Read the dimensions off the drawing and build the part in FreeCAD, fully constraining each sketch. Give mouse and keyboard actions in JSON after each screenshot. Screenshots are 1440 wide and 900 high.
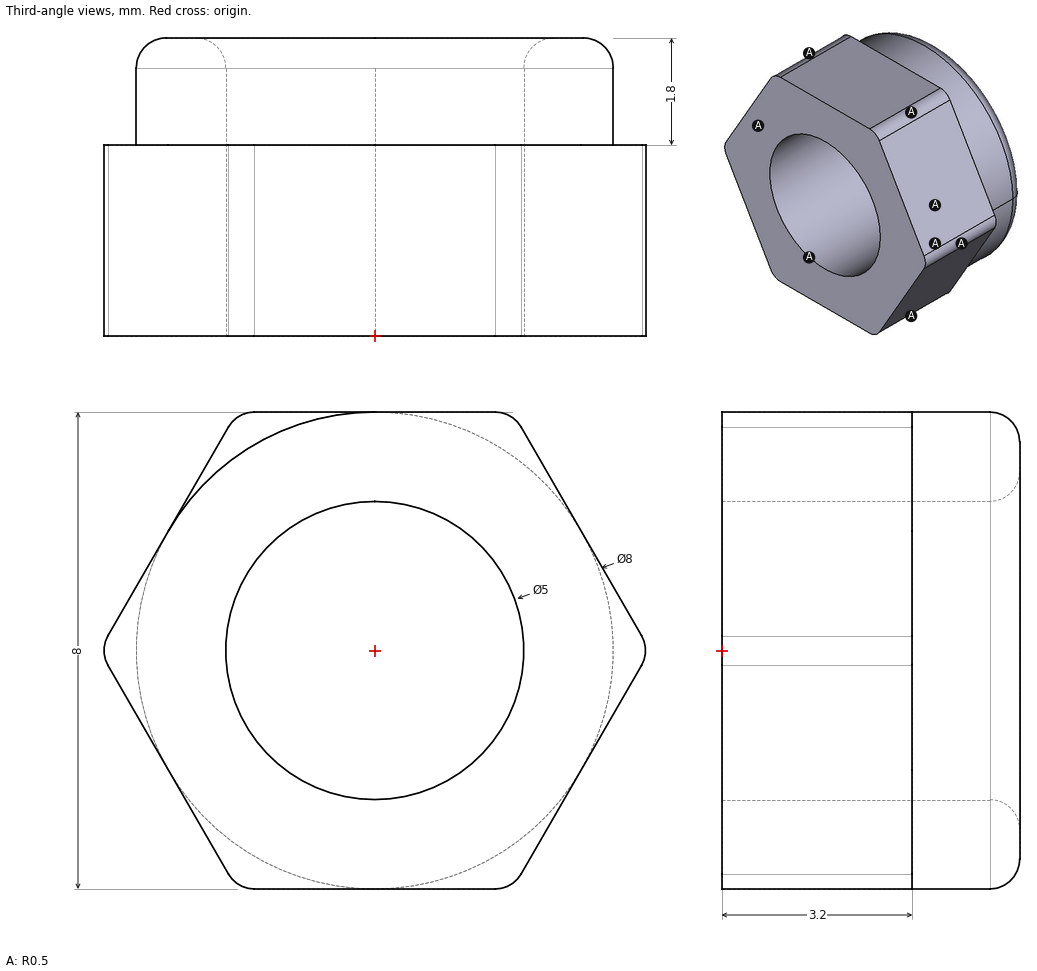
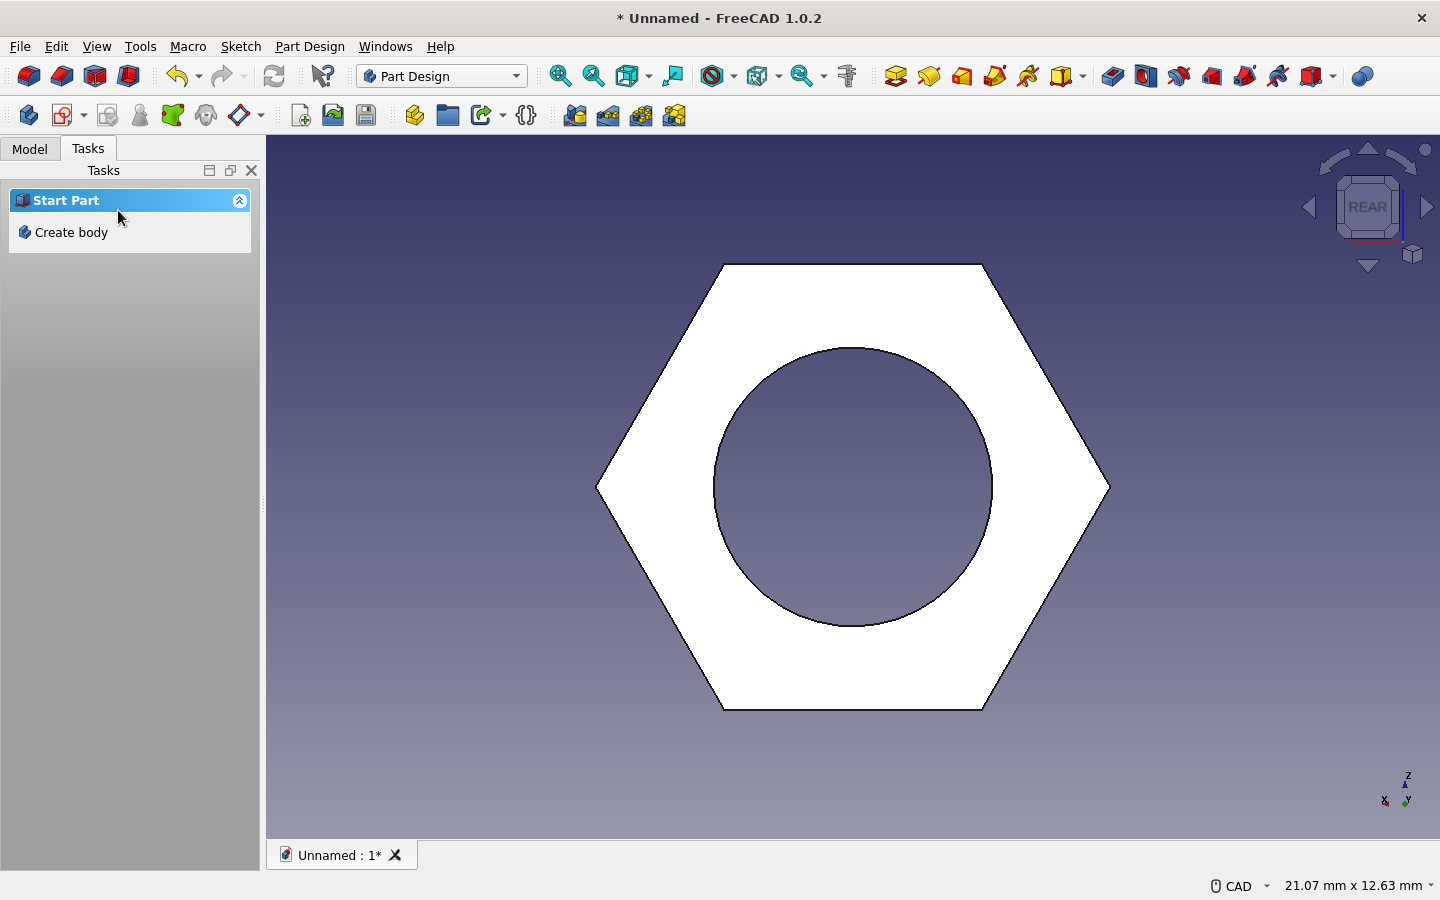
{"action": "left_click", "coordinate": [706, 613]}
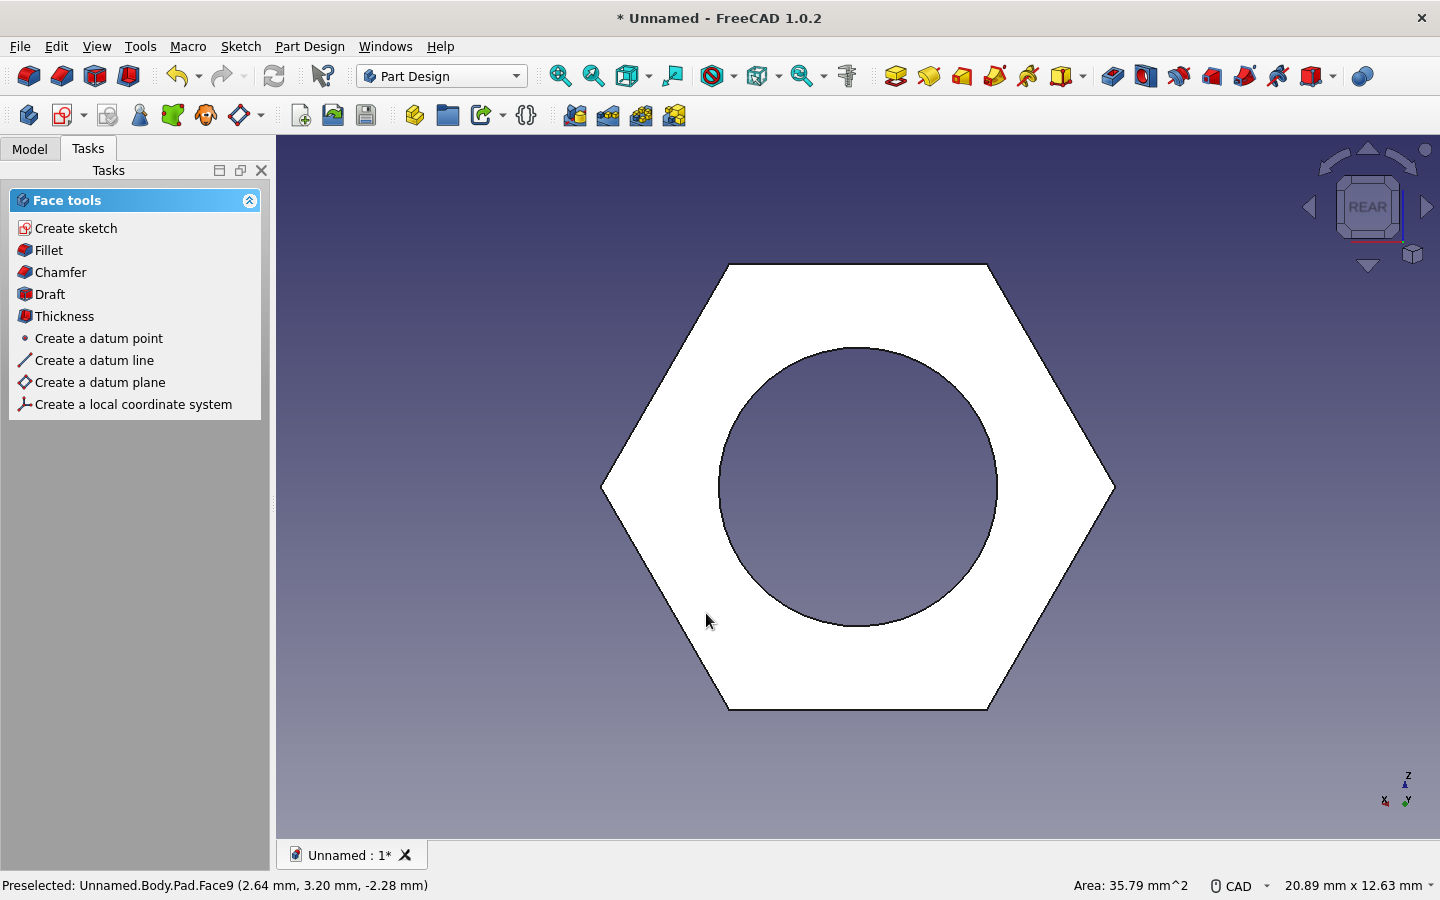
{"action": "left_click", "coordinate": [62, 116]}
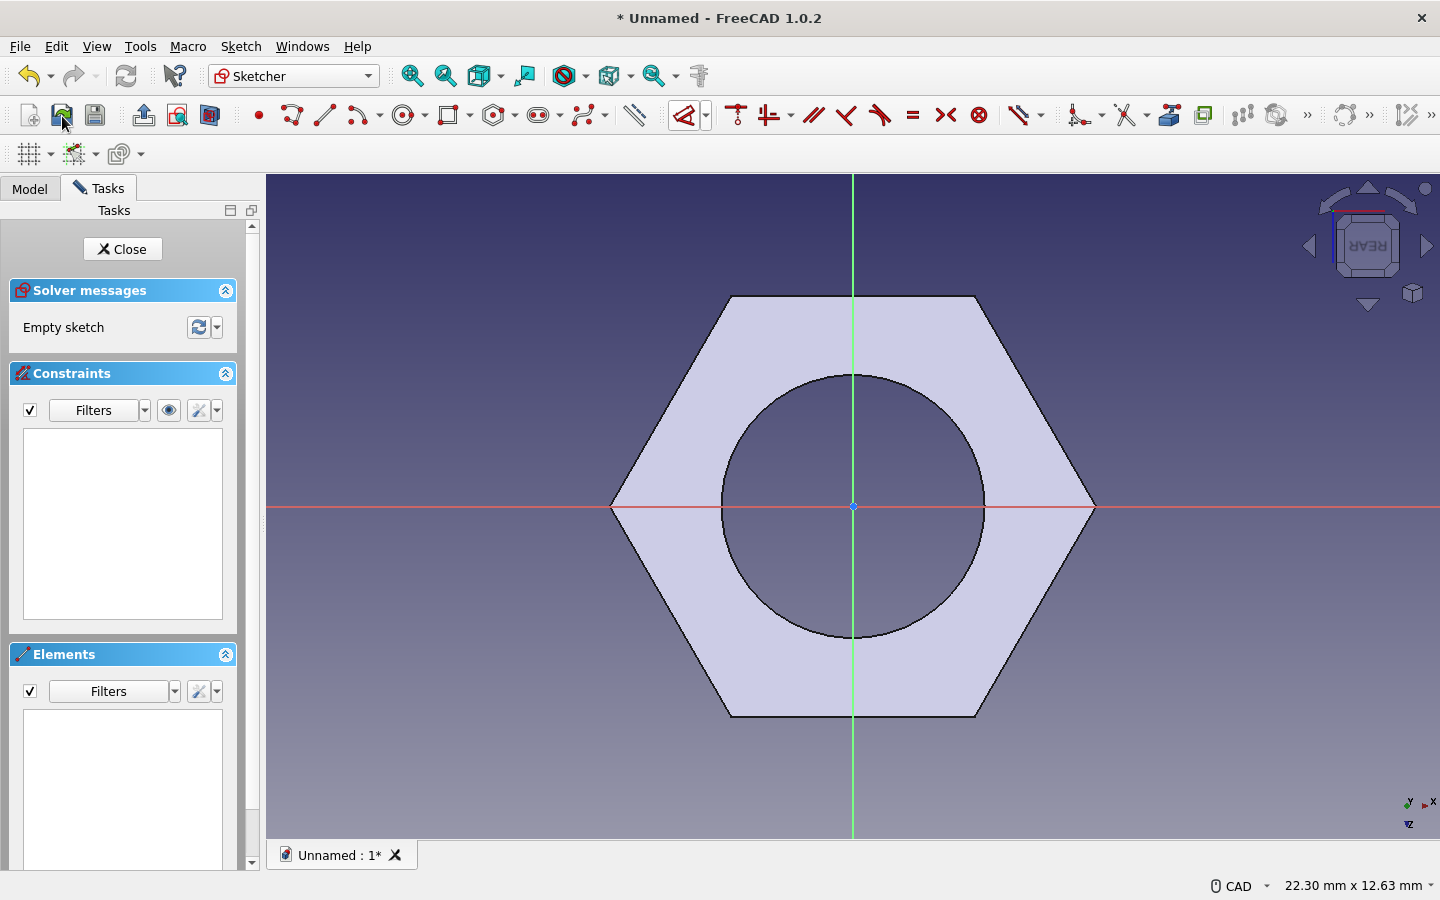
{"action": "left_click", "coordinate": [402, 116]}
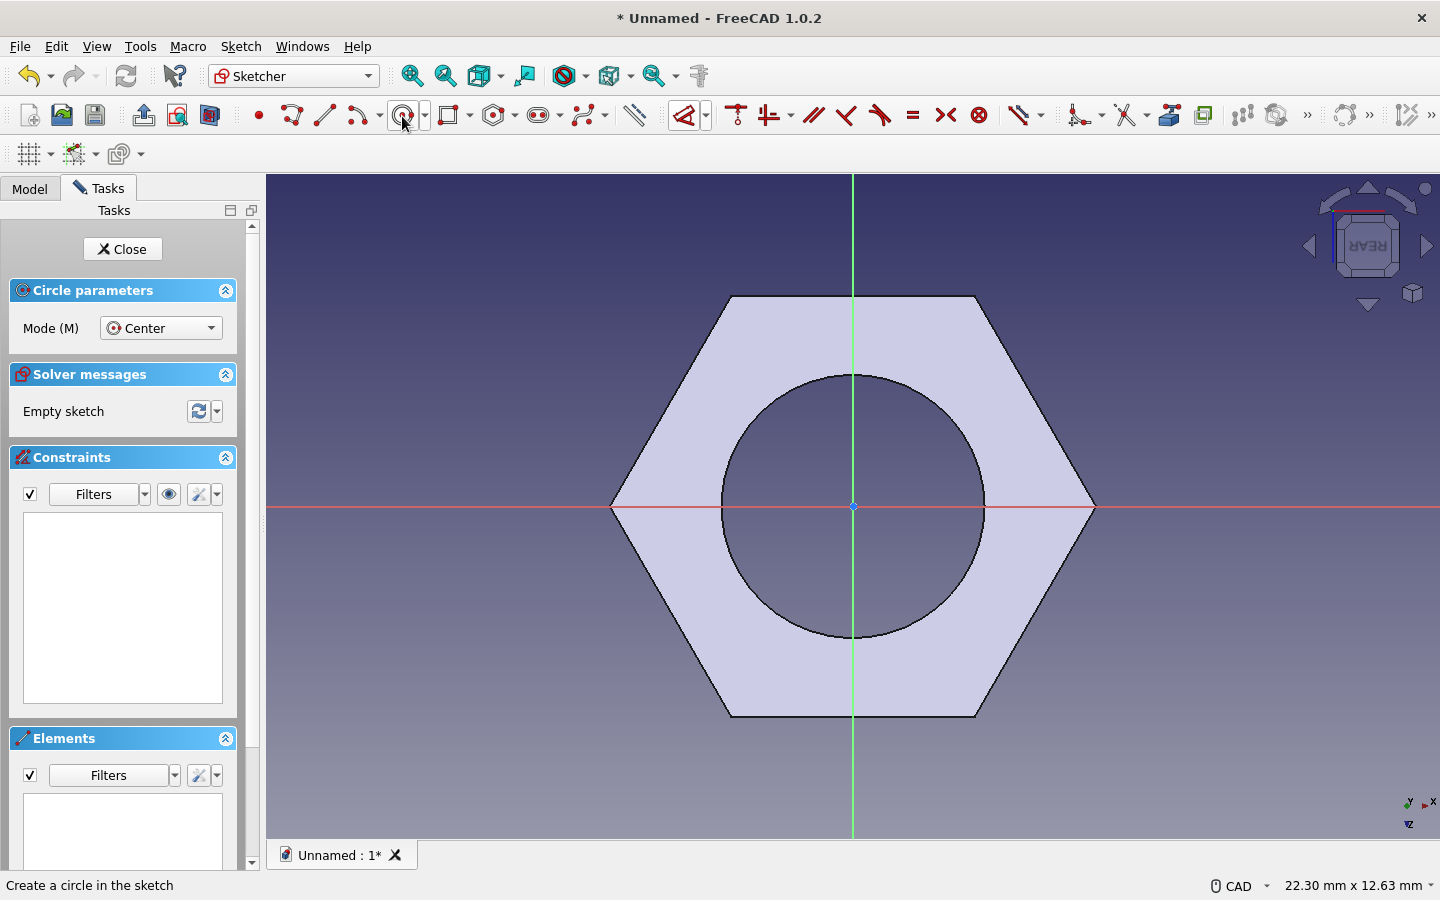
{"action": "left_click", "coordinate": [853, 507]}
{"action": "left_click", "coordinate": [1002, 358]}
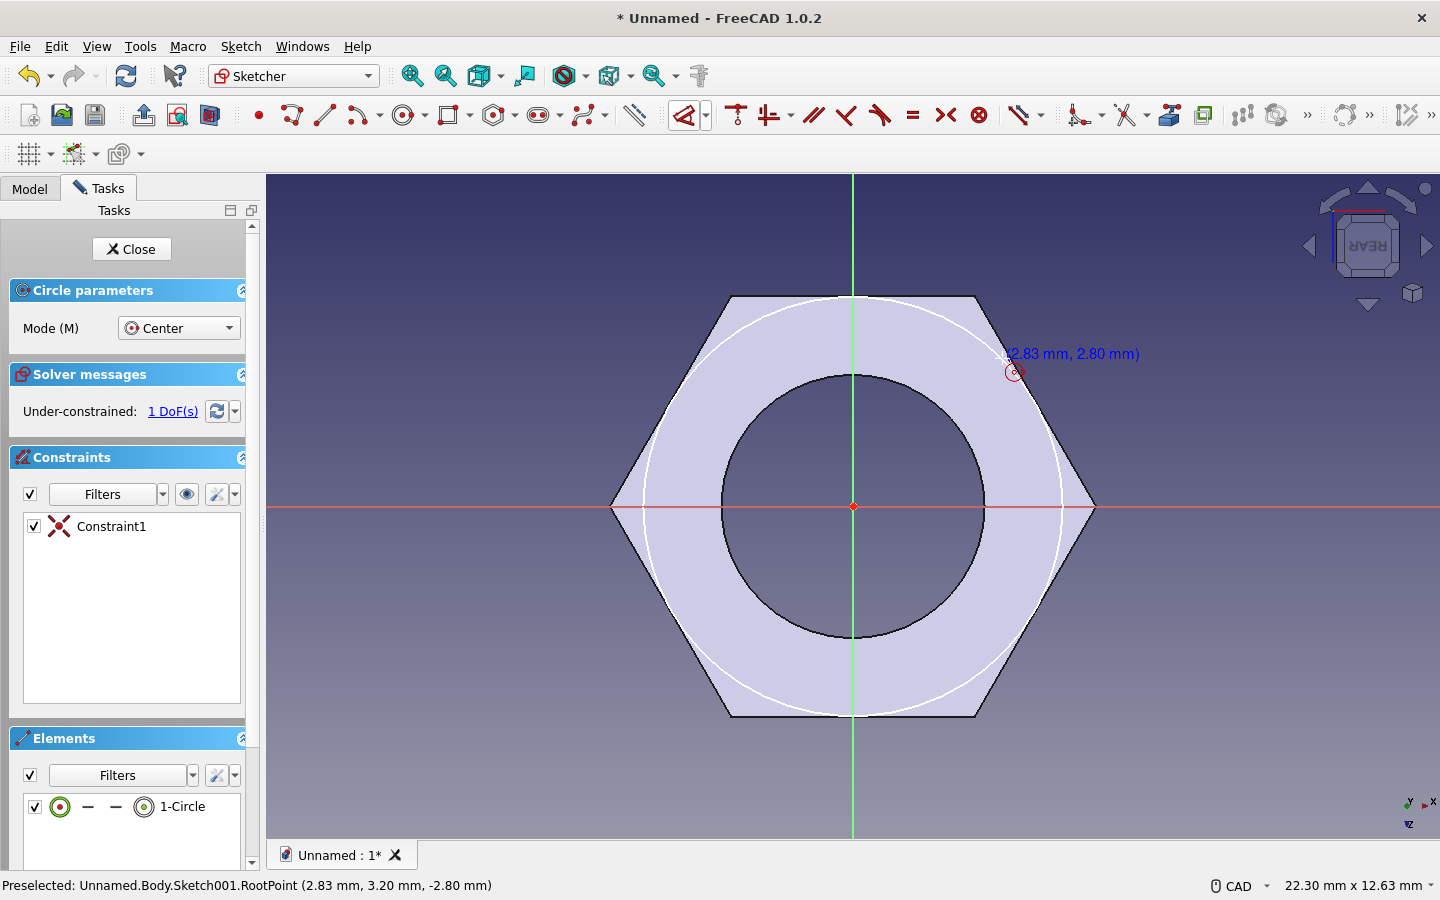
{"action": "left_click", "coordinate": [853, 507]}
{"action": "left_click", "coordinate": [946, 413]}
{"action": "key", "text": "Escape"}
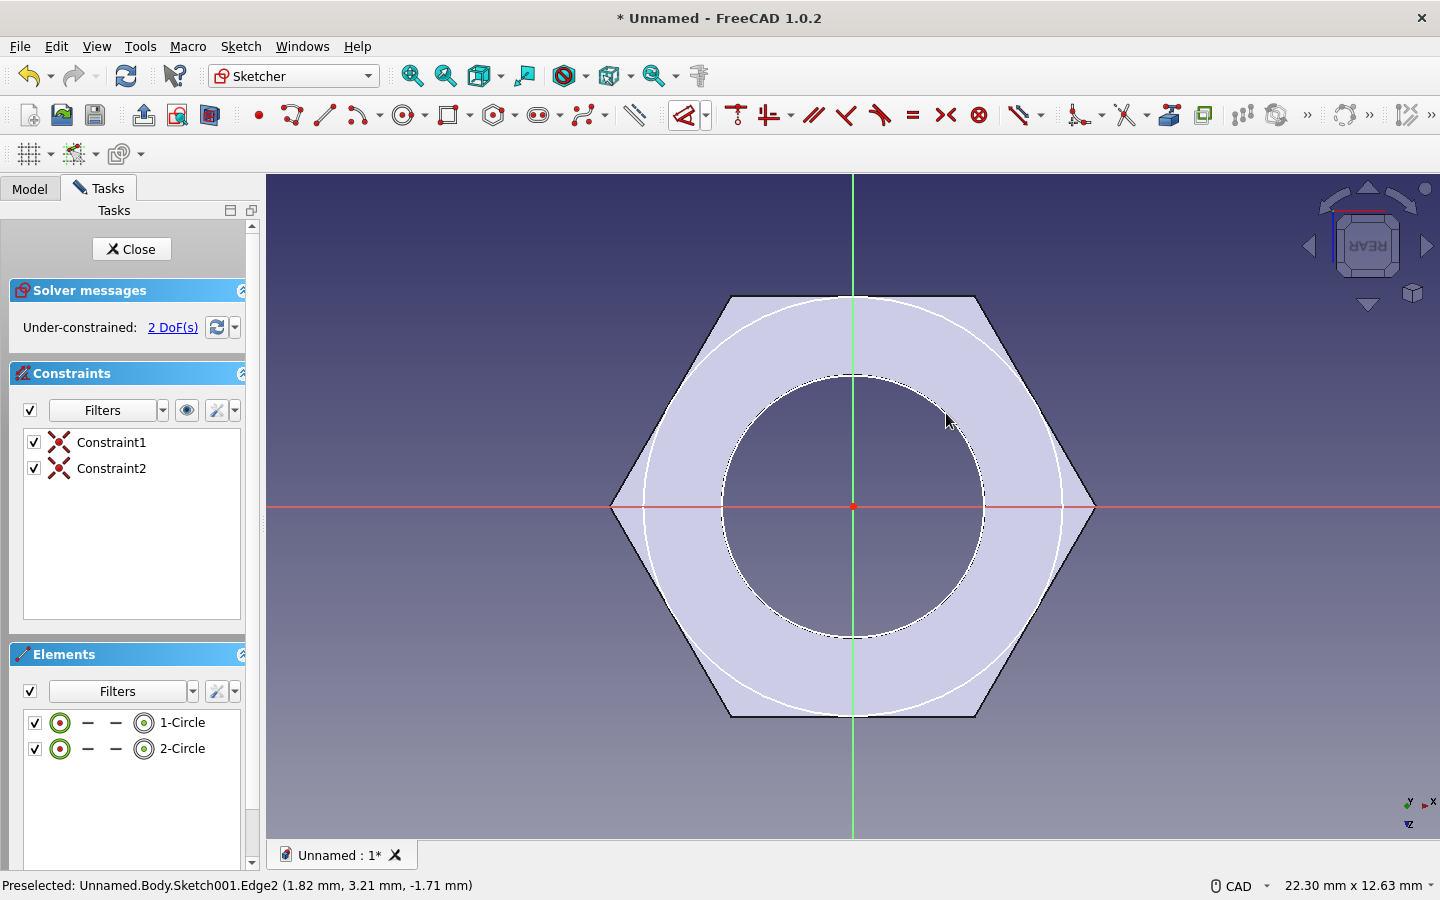
{"action": "left_click", "coordinate": [1001, 358]}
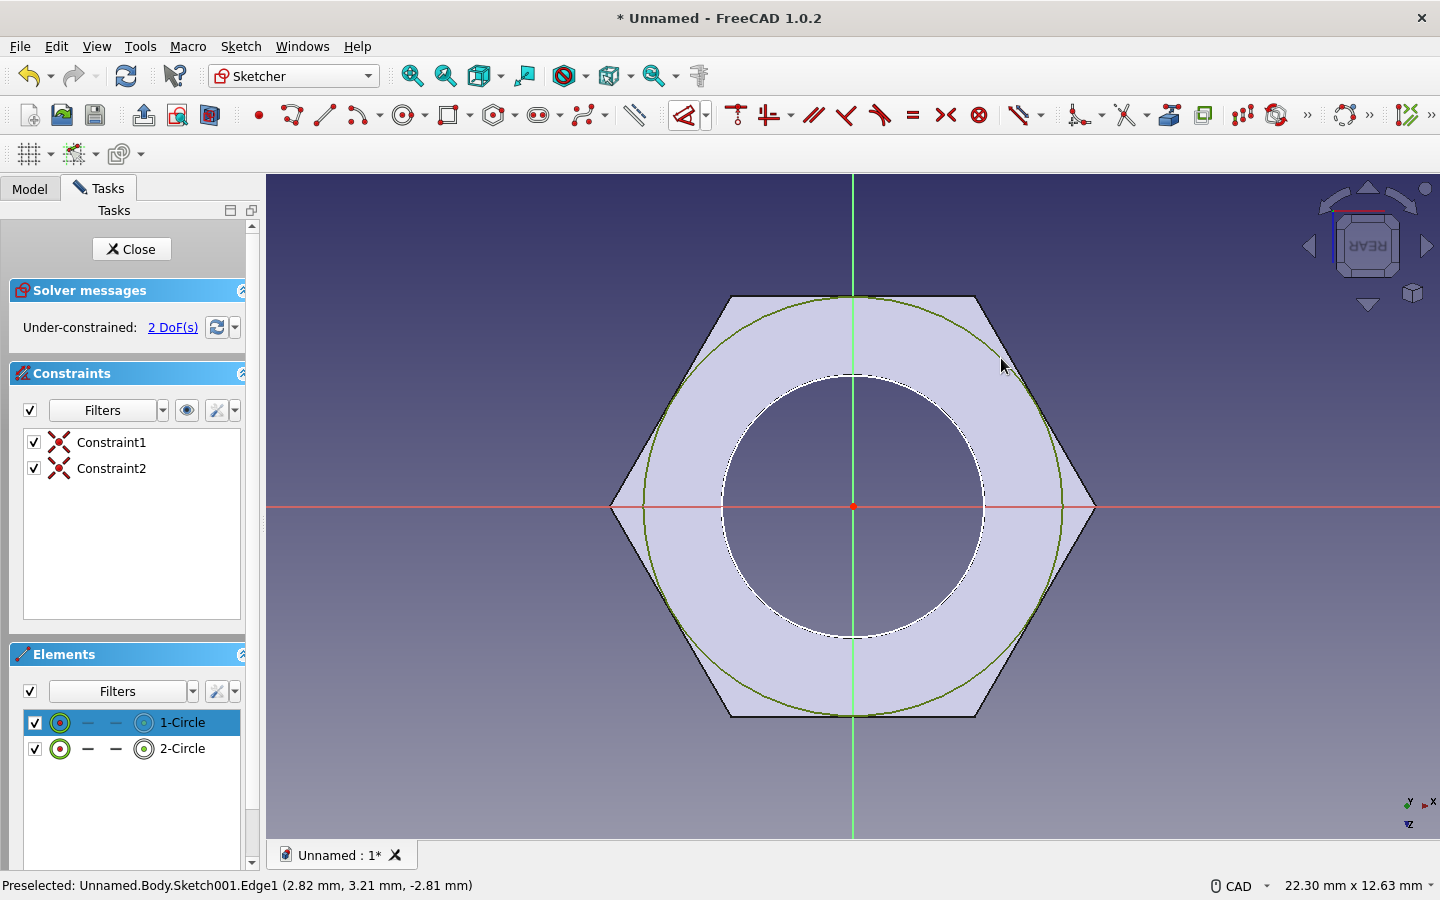
{"action": "left_click", "coordinate": [706, 116]}